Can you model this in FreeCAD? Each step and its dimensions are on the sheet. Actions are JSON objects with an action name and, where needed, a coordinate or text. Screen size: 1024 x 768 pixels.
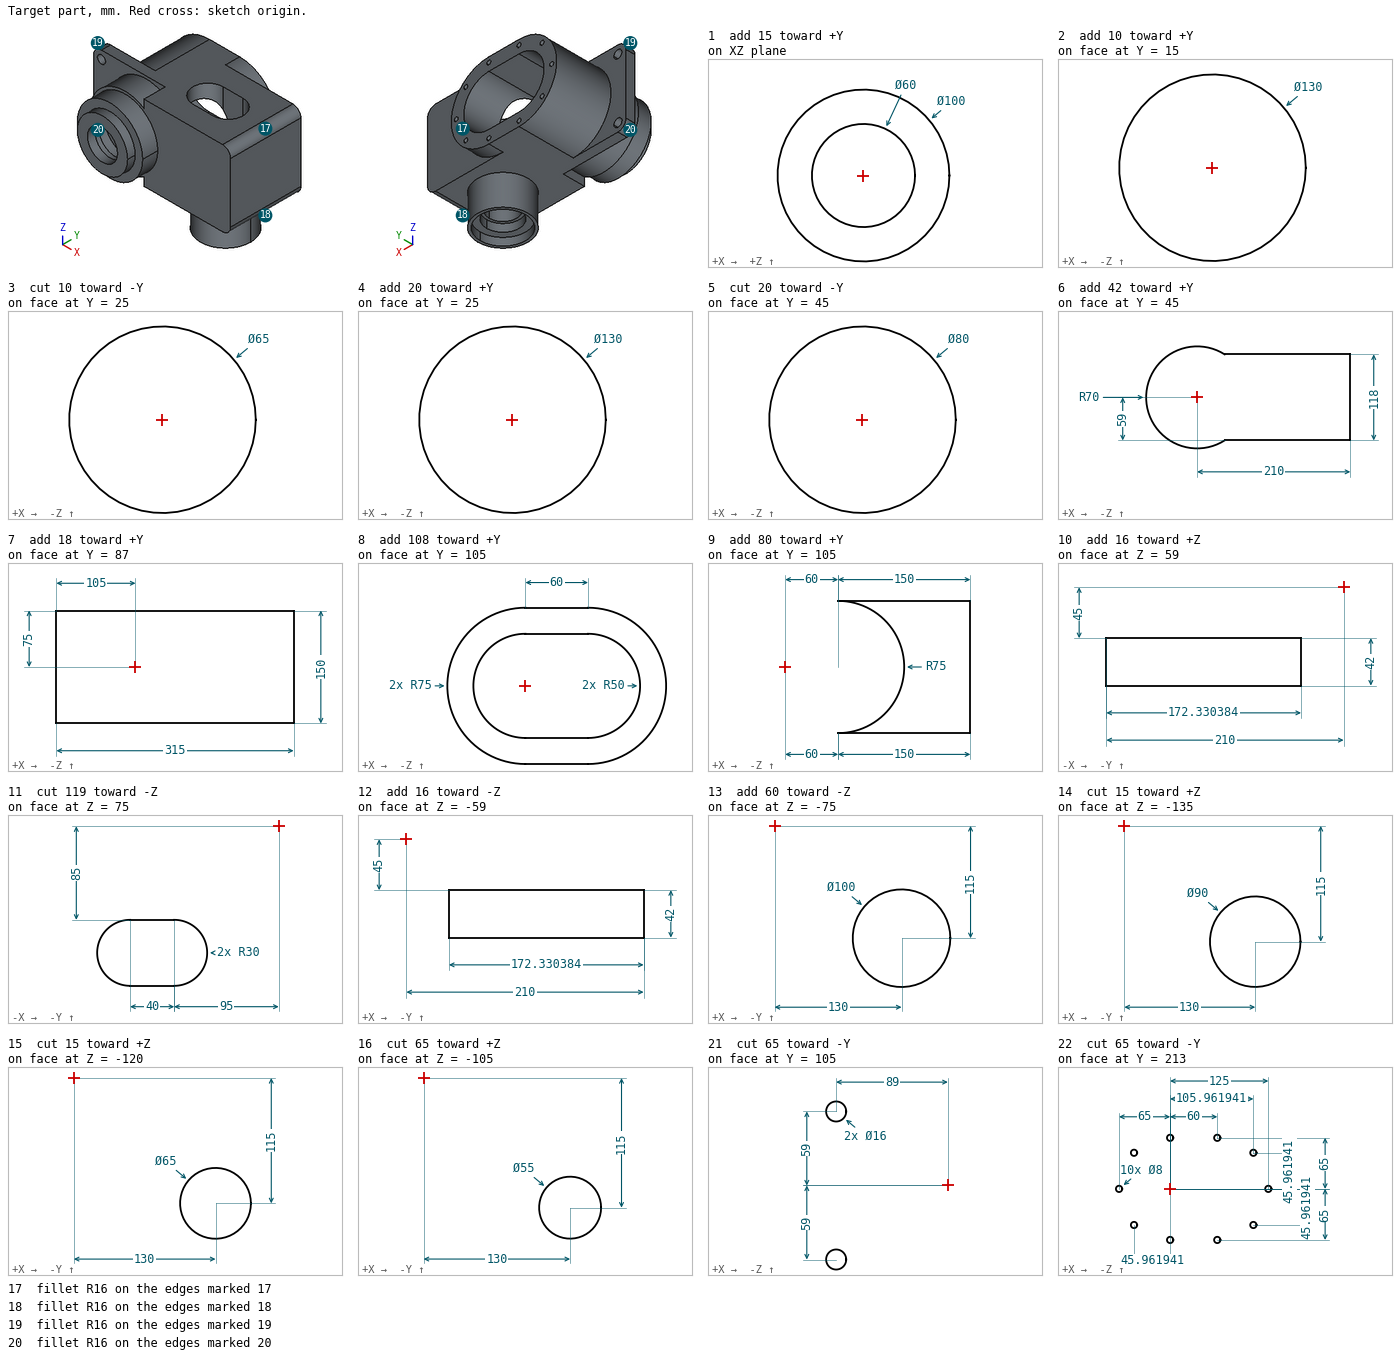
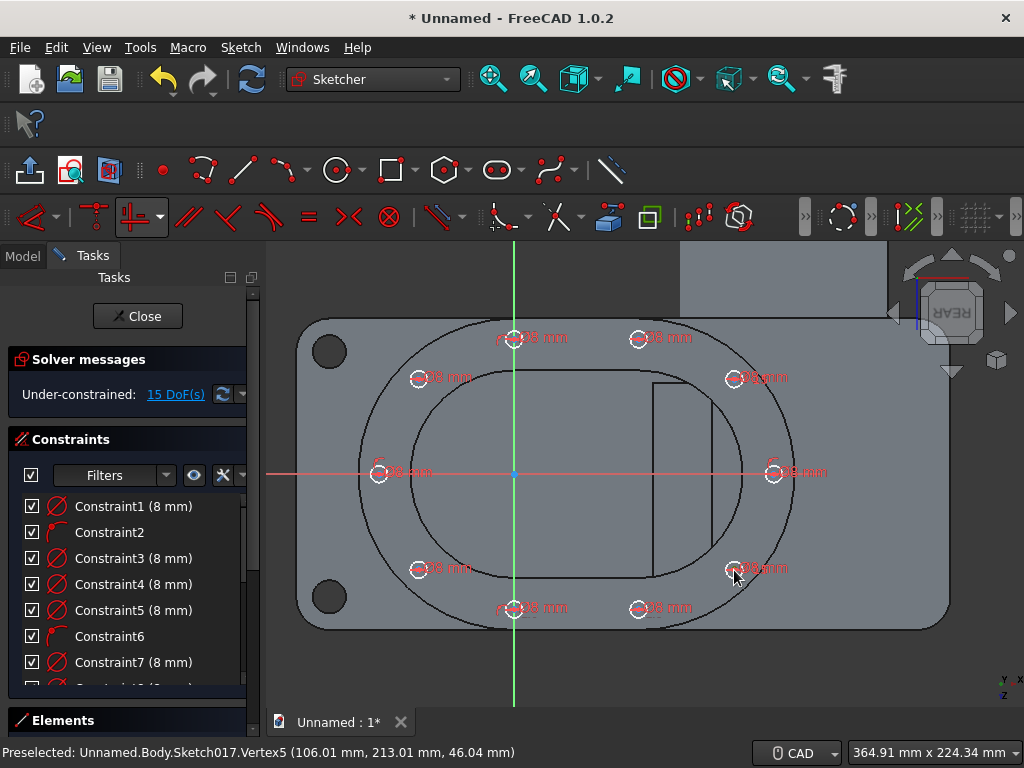
{"action": "left_click", "coordinate": [419, 570]}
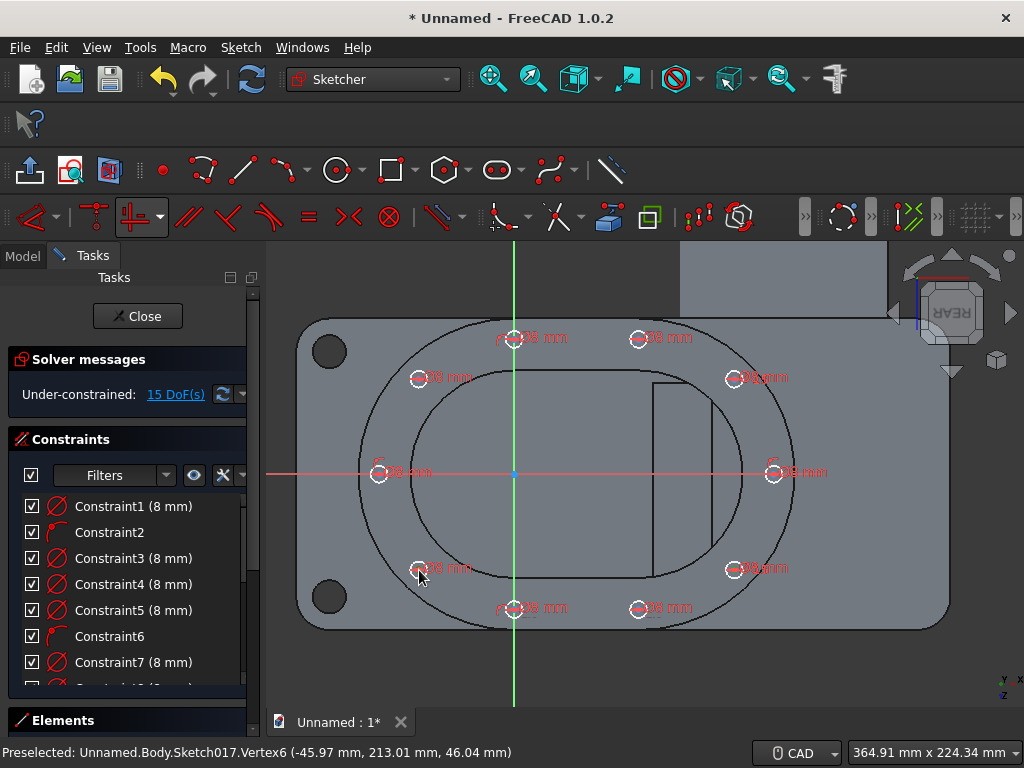
{"action": "key", "text": "h"}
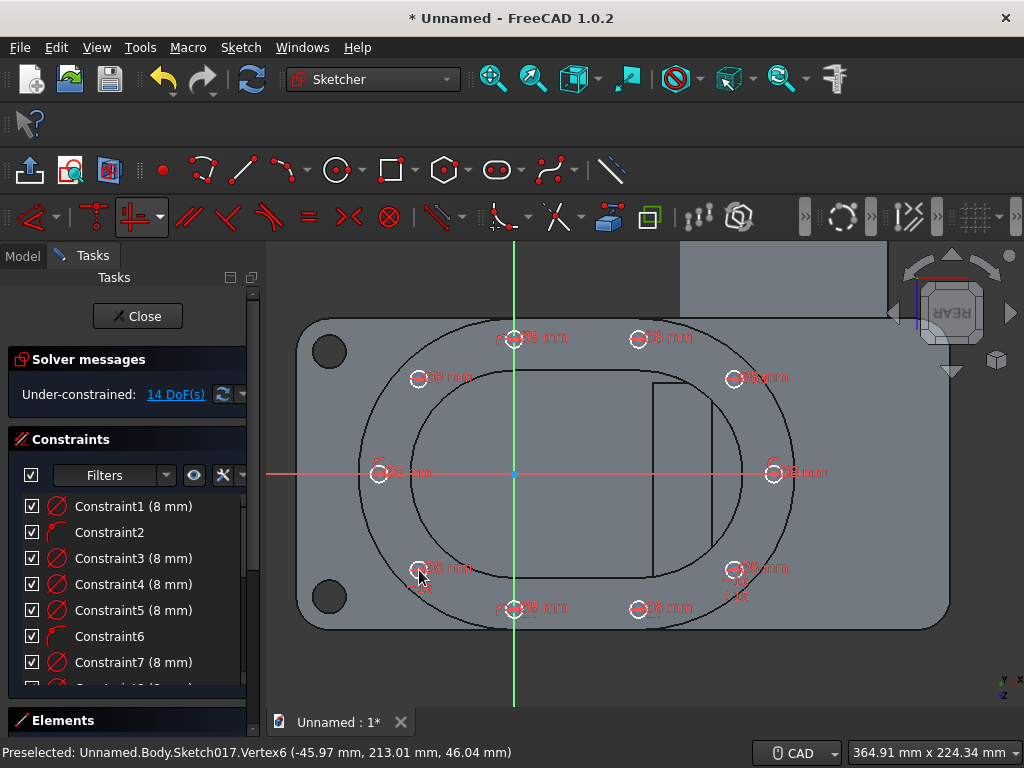
{"action": "left_click", "coordinate": [419, 570]}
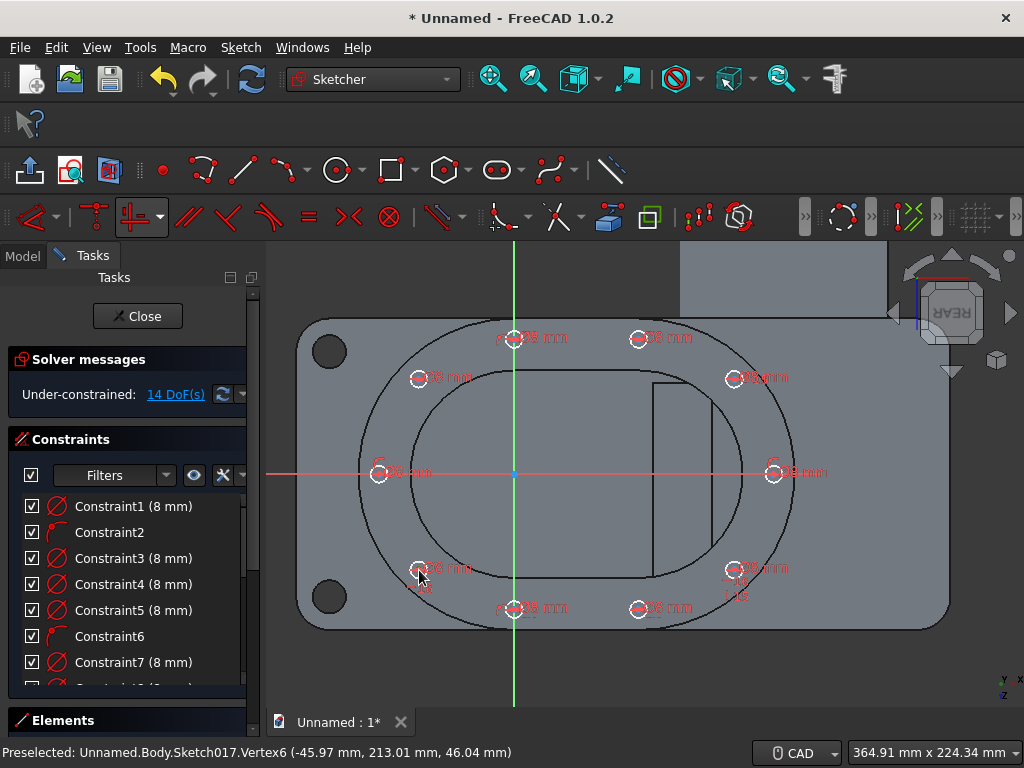
{"action": "left_click", "coordinate": [419, 379]}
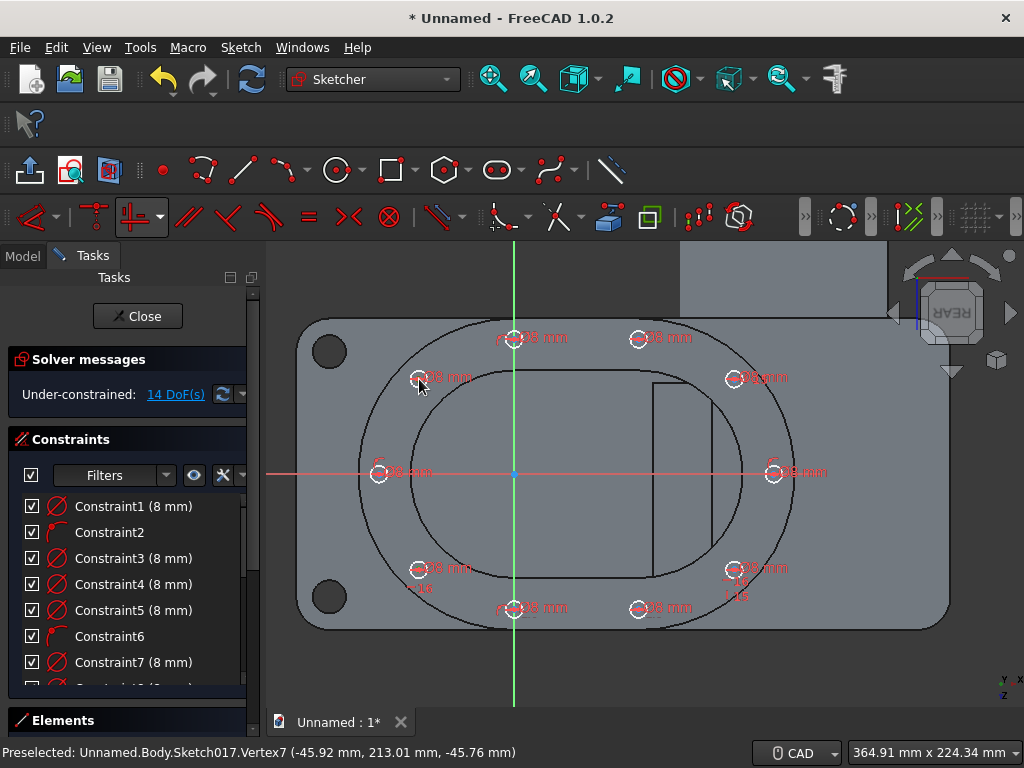
{"action": "left_click", "coordinate": [162, 218]}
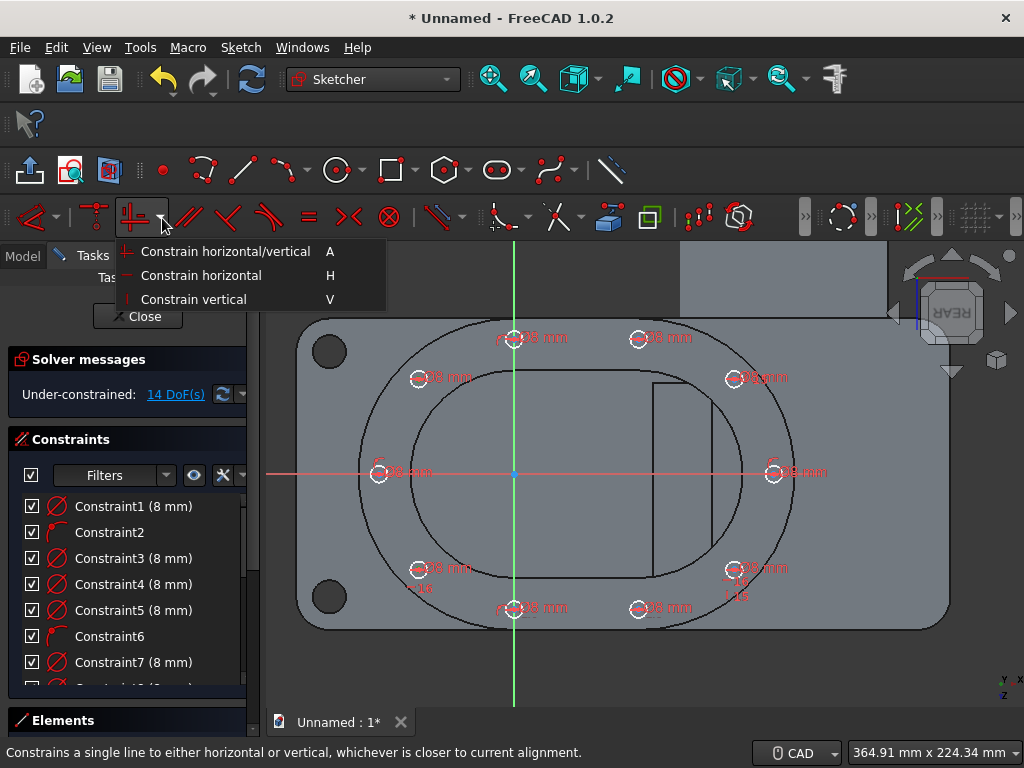
{"action": "left_click", "coordinate": [251, 299]}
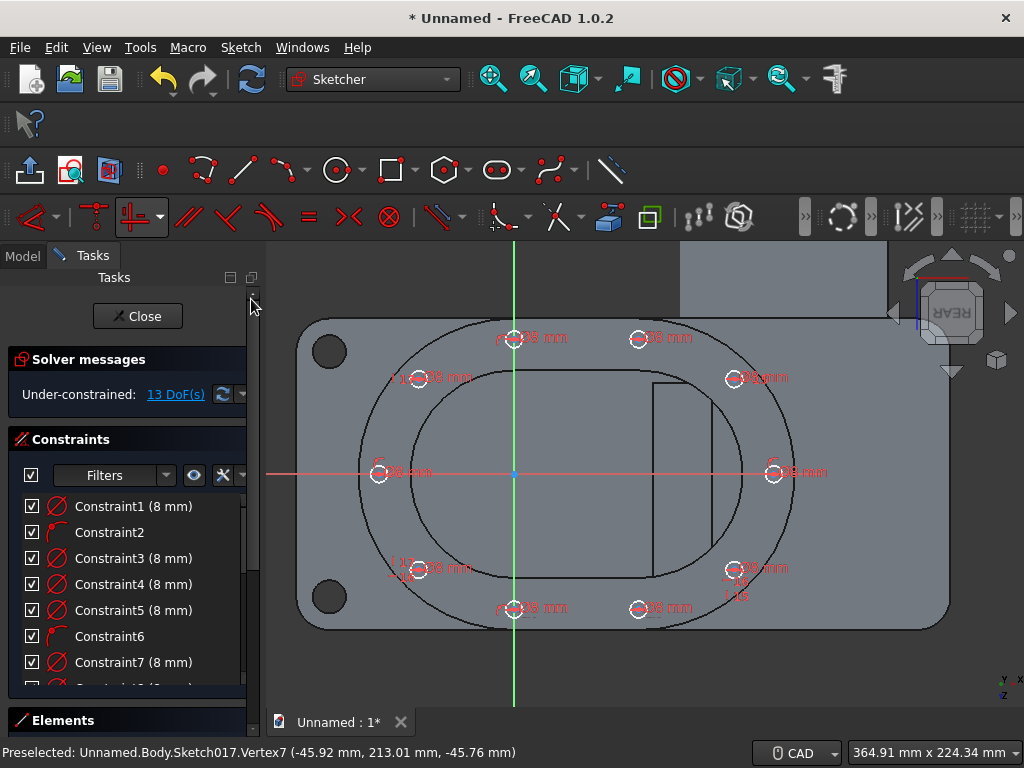
{"action": "left_click", "coordinate": [734, 379]}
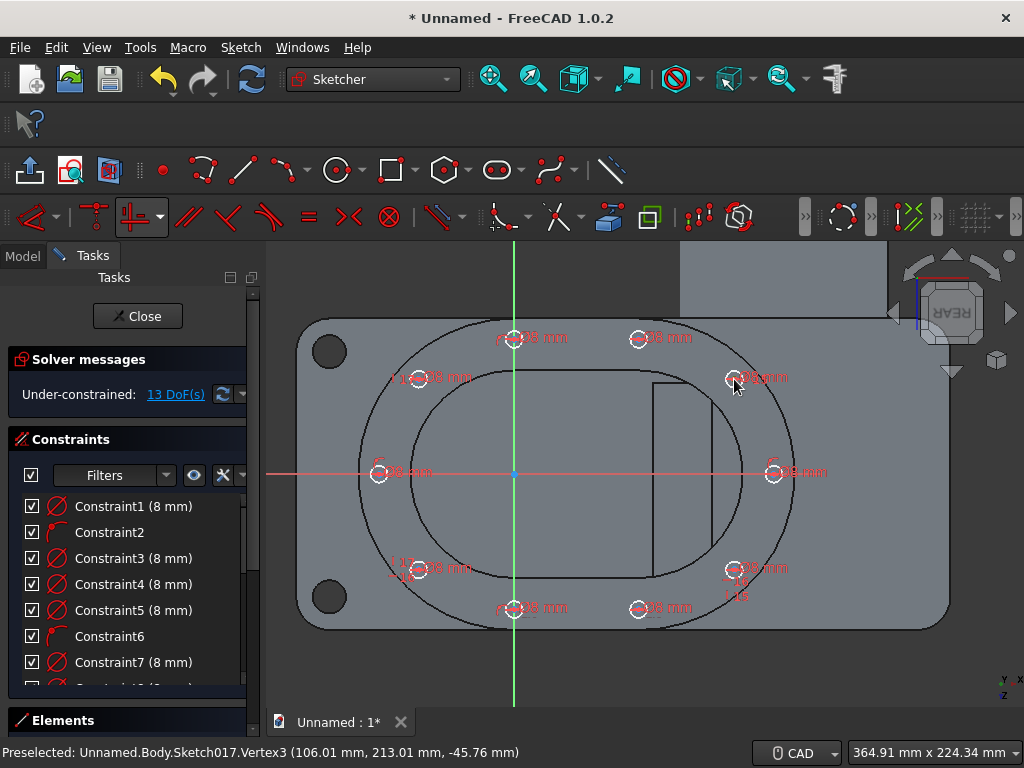
{"action": "left_click", "coordinate": [419, 379]}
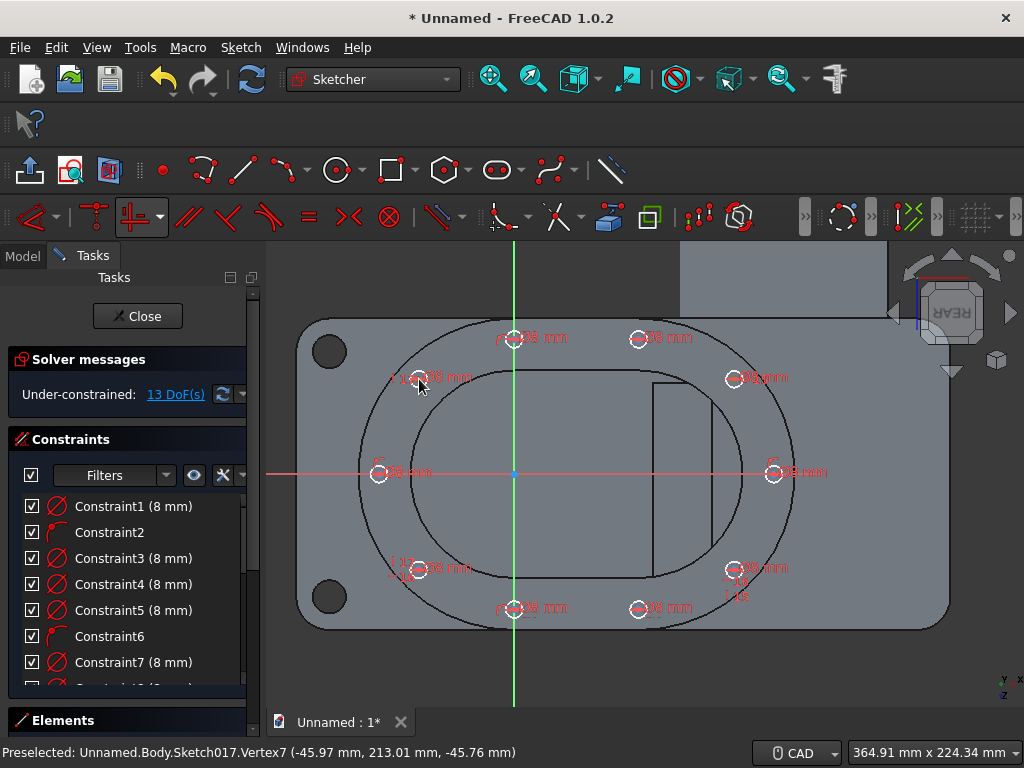
{"action": "key", "text": "h"}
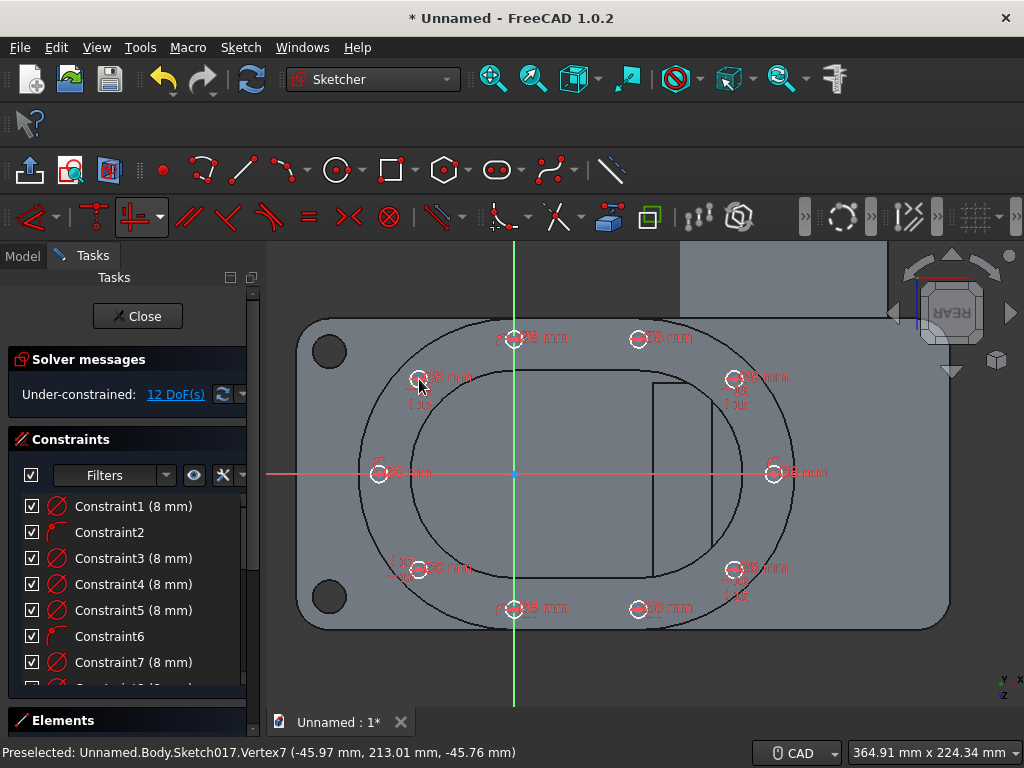
{"action": "left_click", "coordinate": [639, 339]}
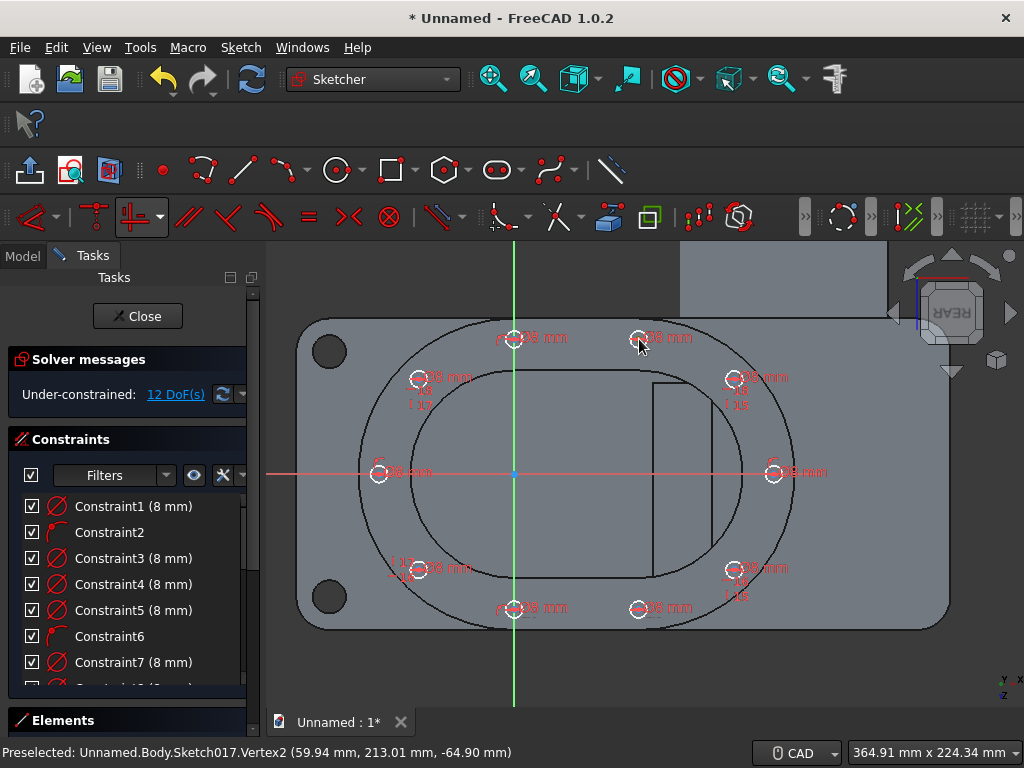
{"action": "left_click", "coordinate": [514, 339]}